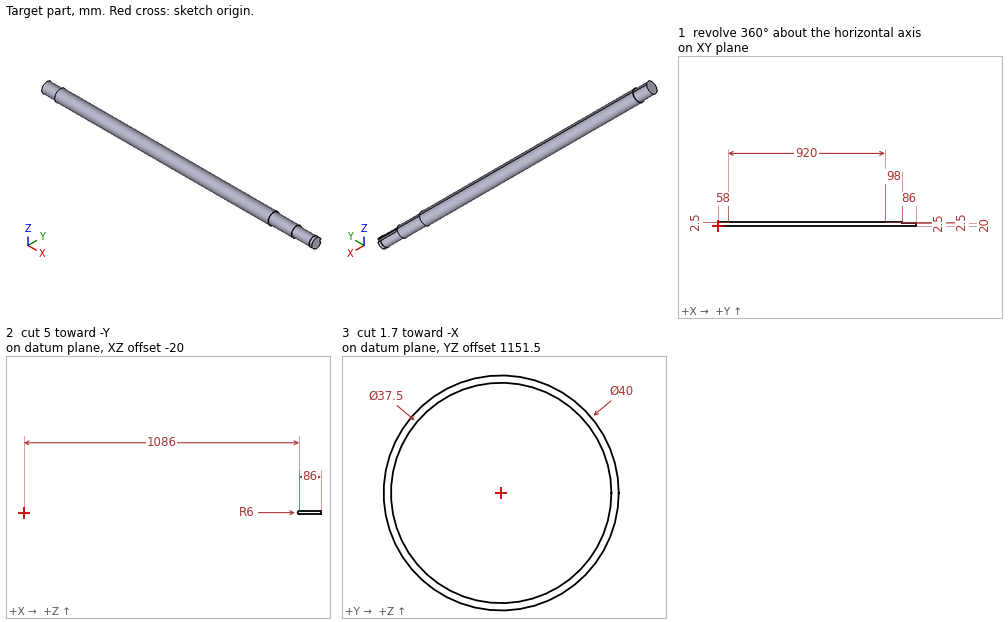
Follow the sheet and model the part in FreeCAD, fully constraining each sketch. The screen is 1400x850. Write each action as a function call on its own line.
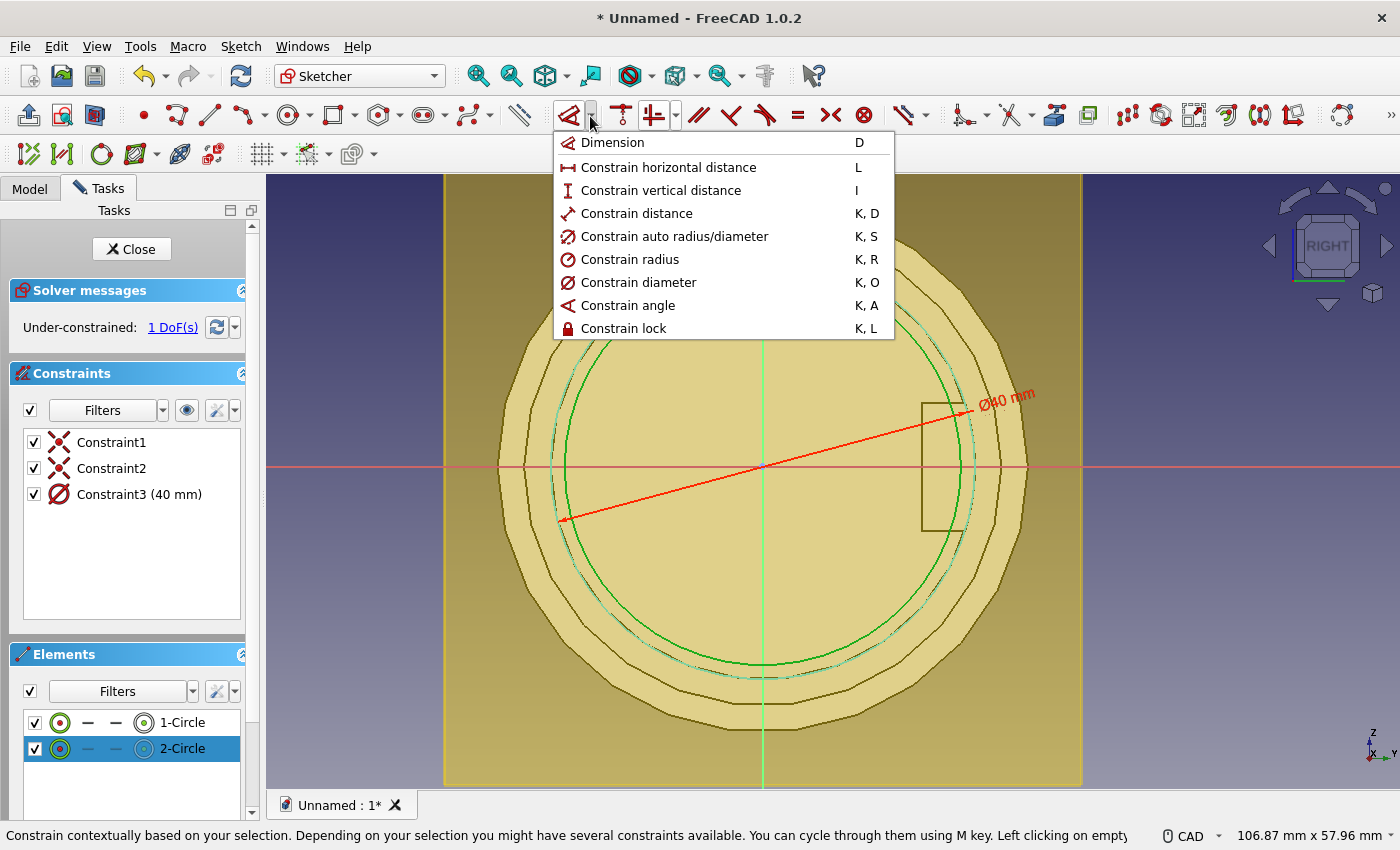
click(724, 282)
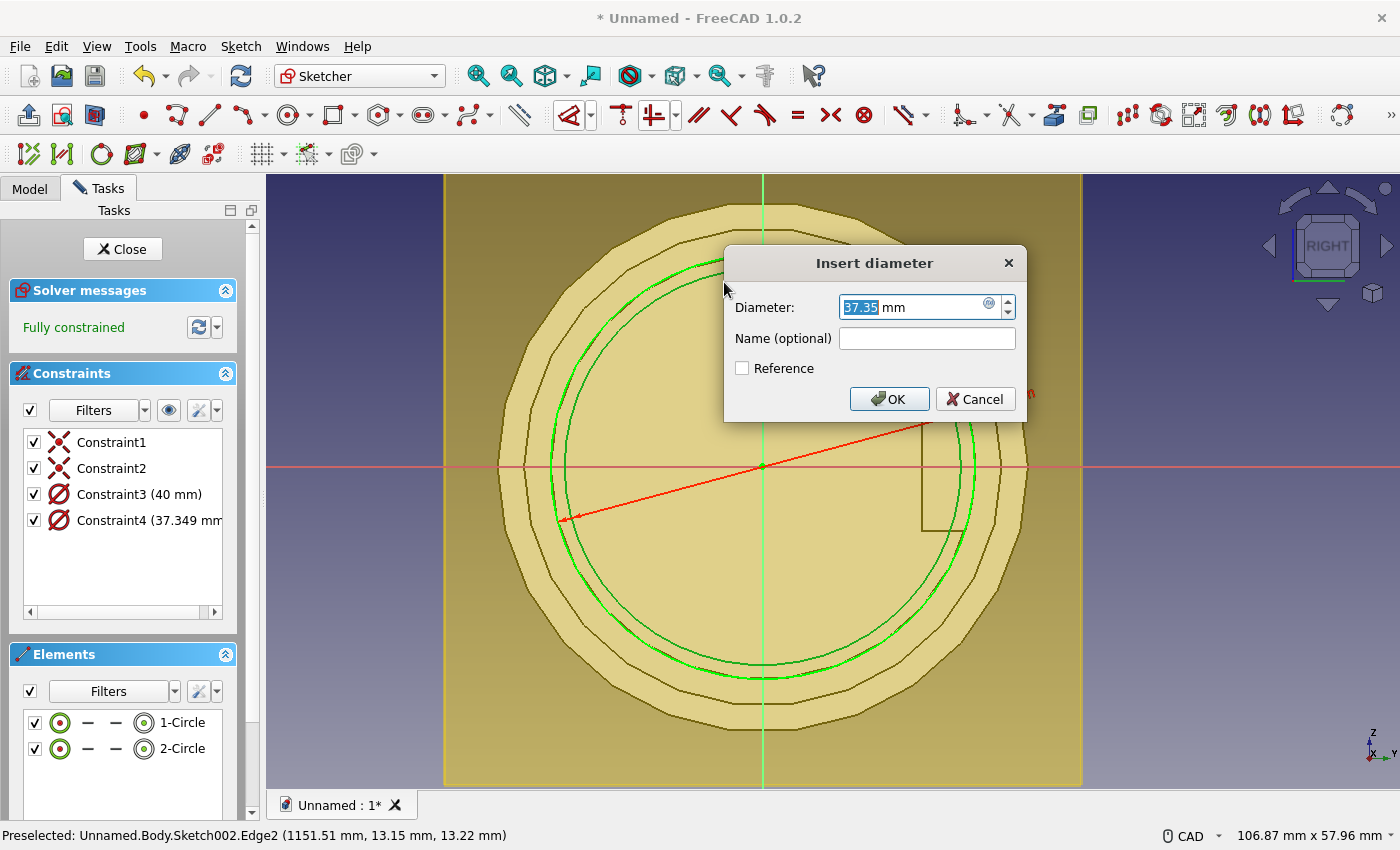
text(37.5)
key(Return)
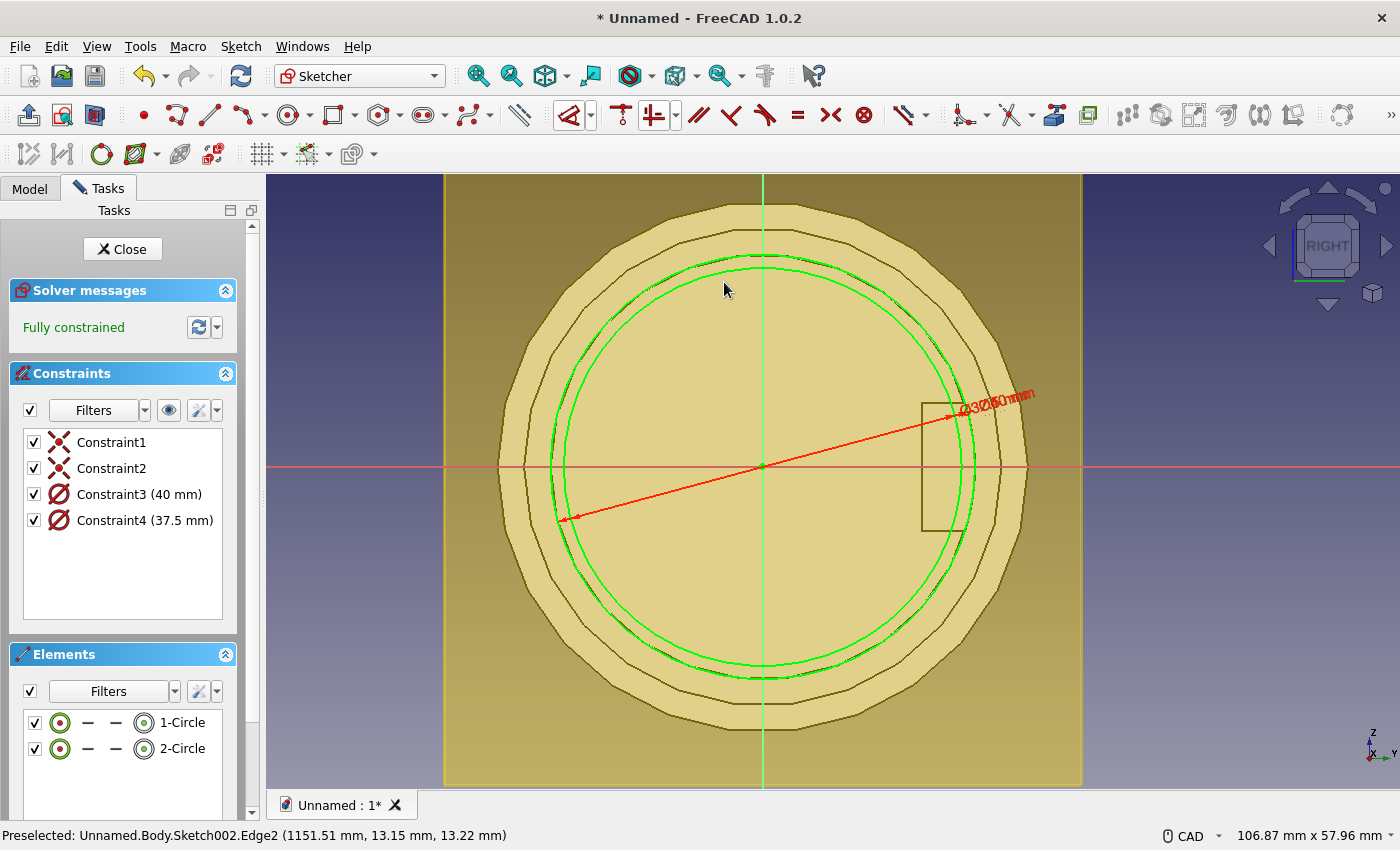
click(123, 249)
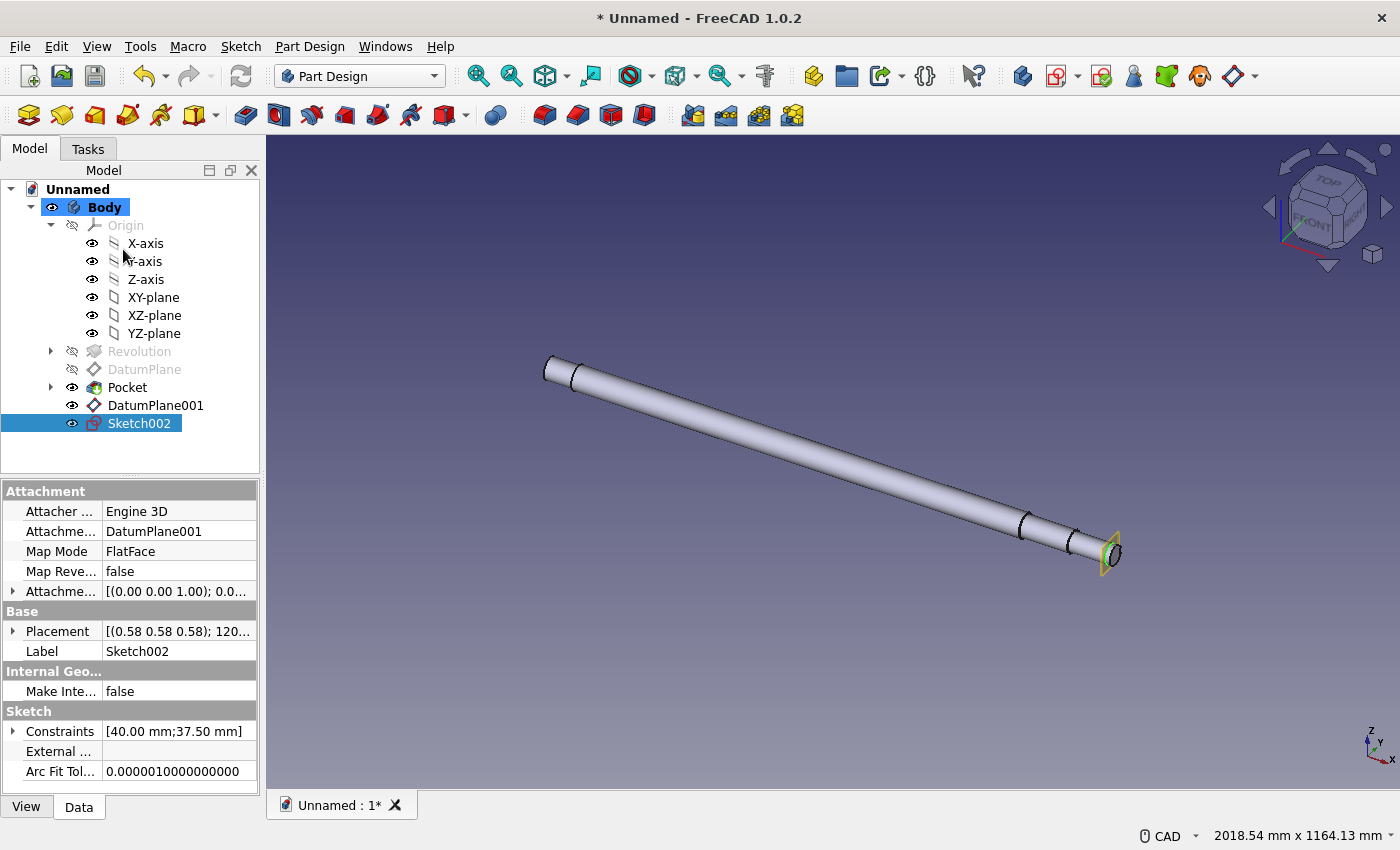
click(246, 116)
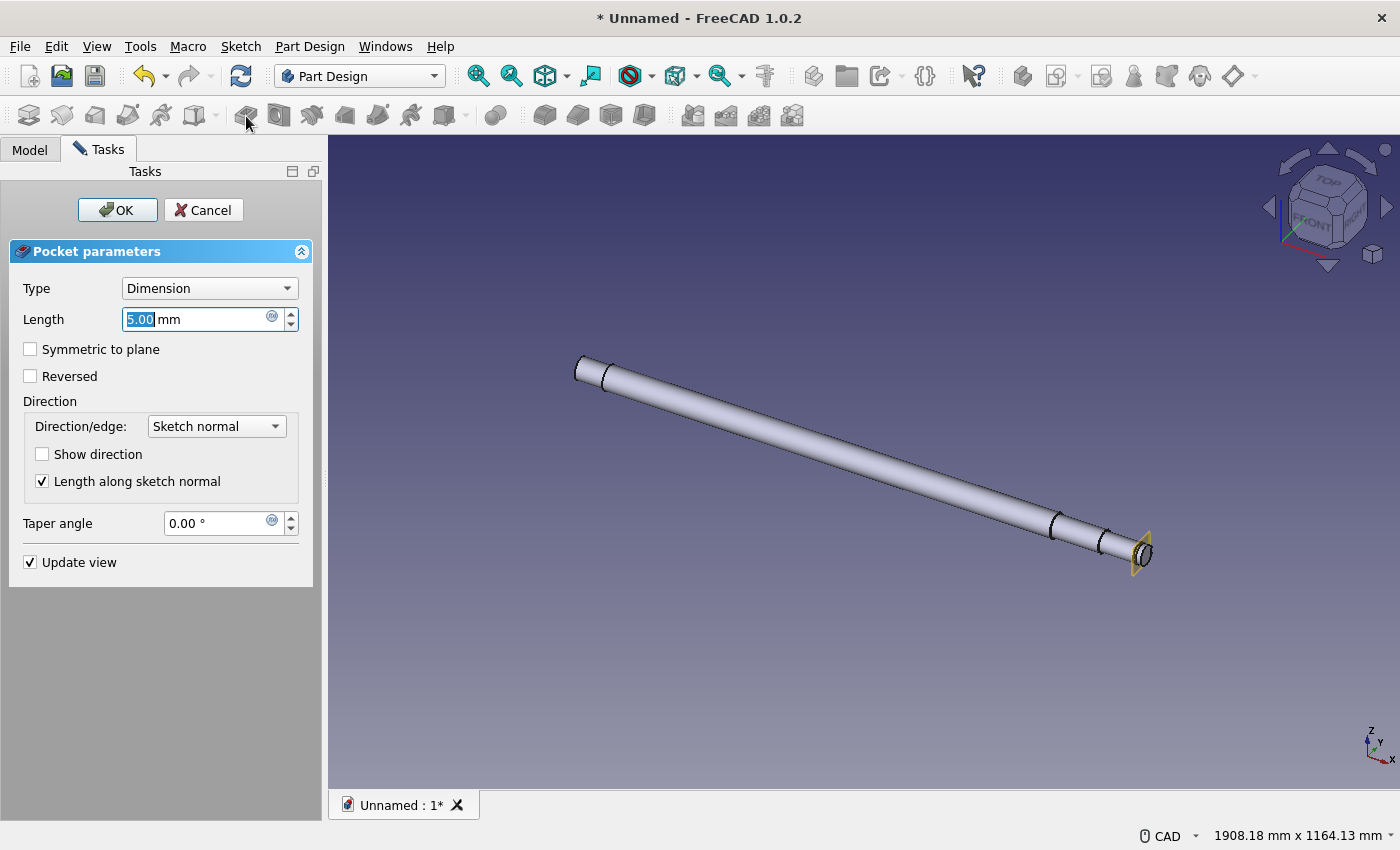
text(1.7)
key(Tab)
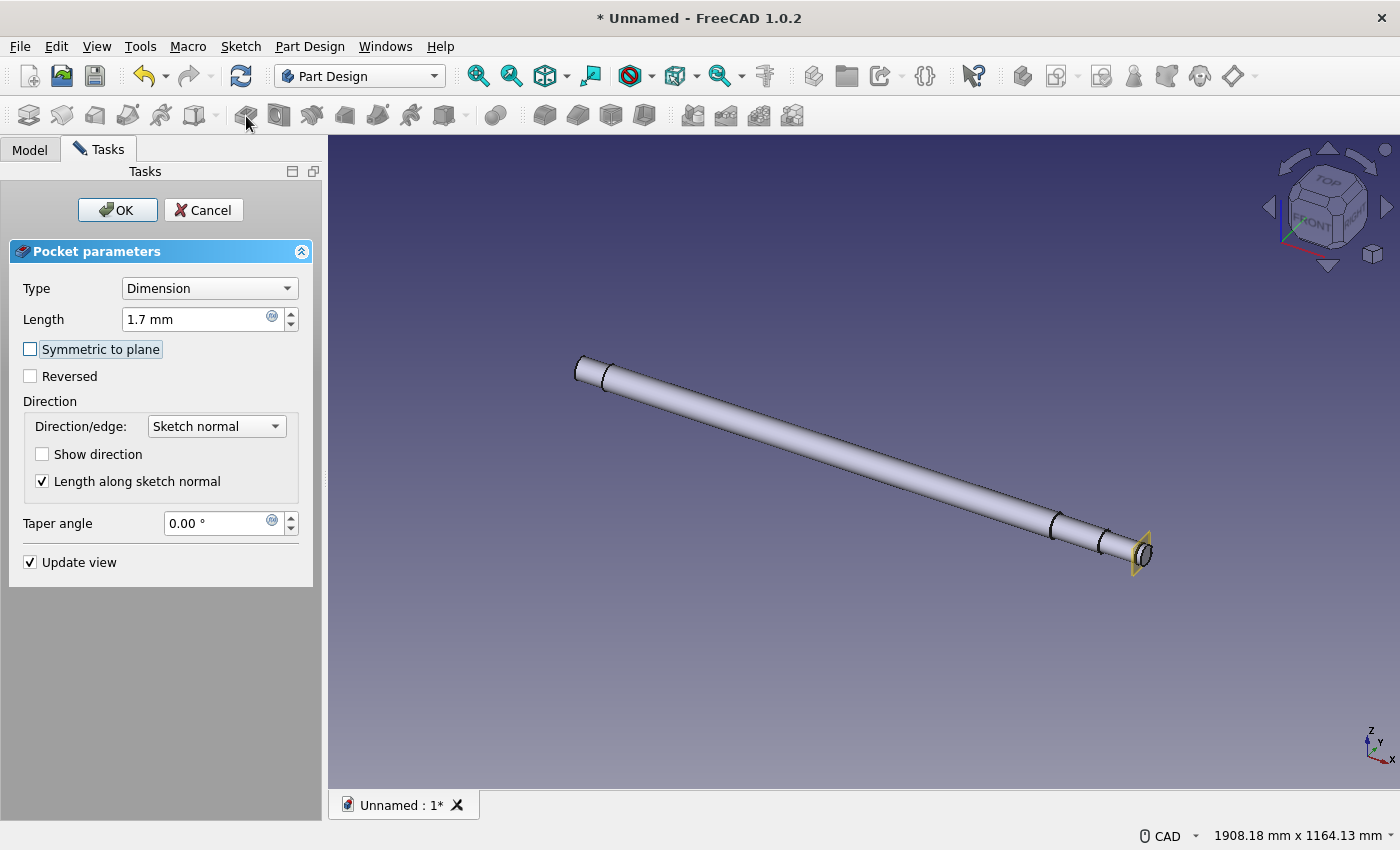
click(118, 210)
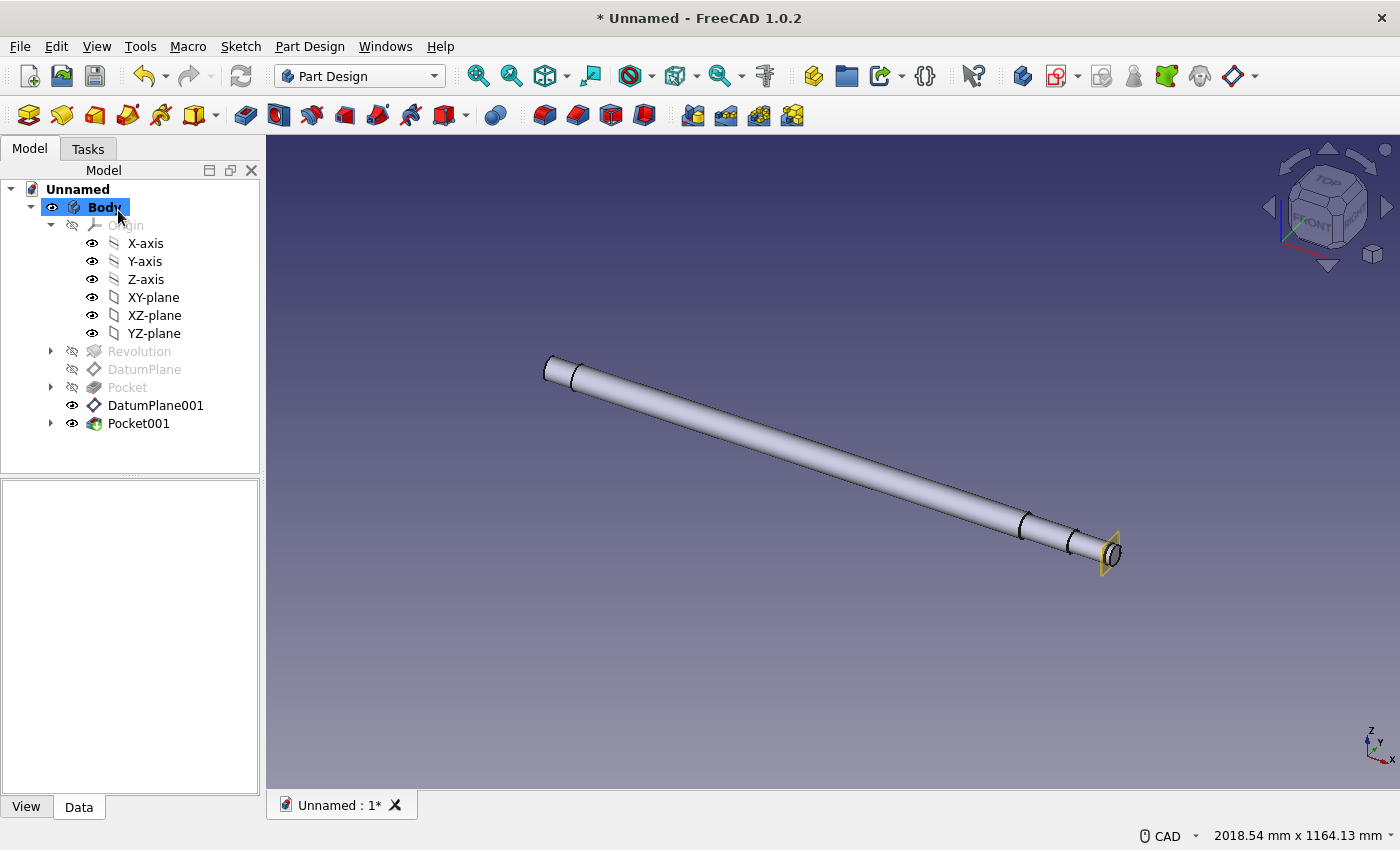
click(117, 405)
key(space)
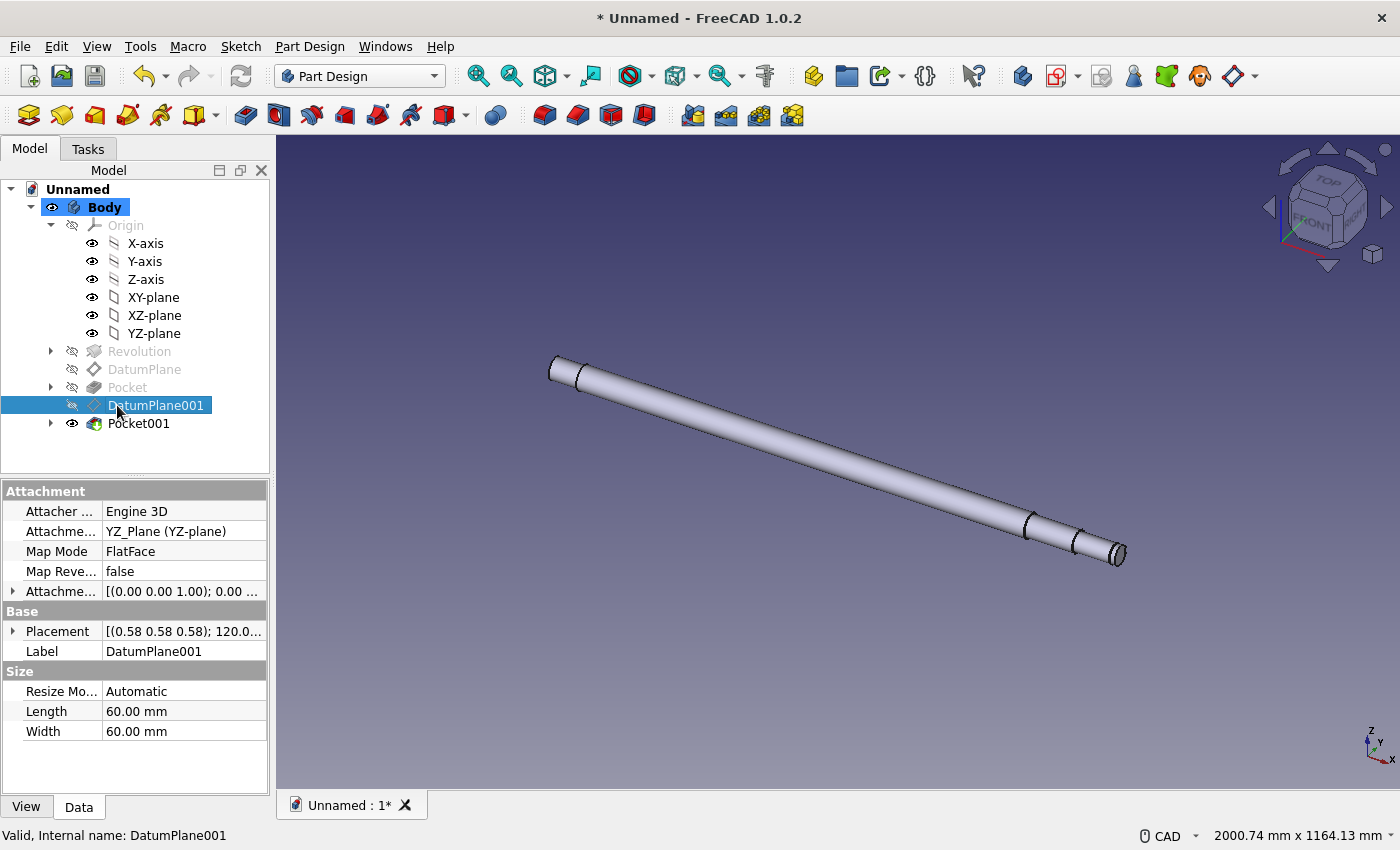
key(0)